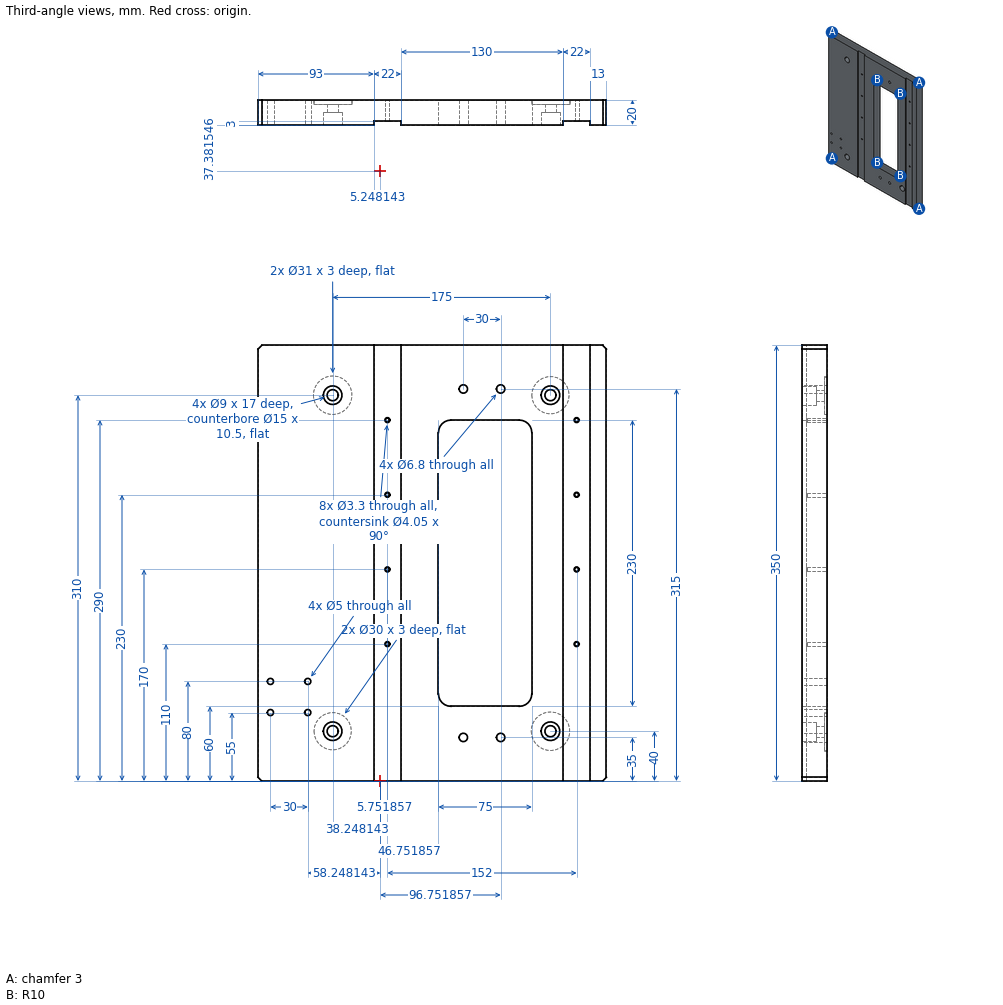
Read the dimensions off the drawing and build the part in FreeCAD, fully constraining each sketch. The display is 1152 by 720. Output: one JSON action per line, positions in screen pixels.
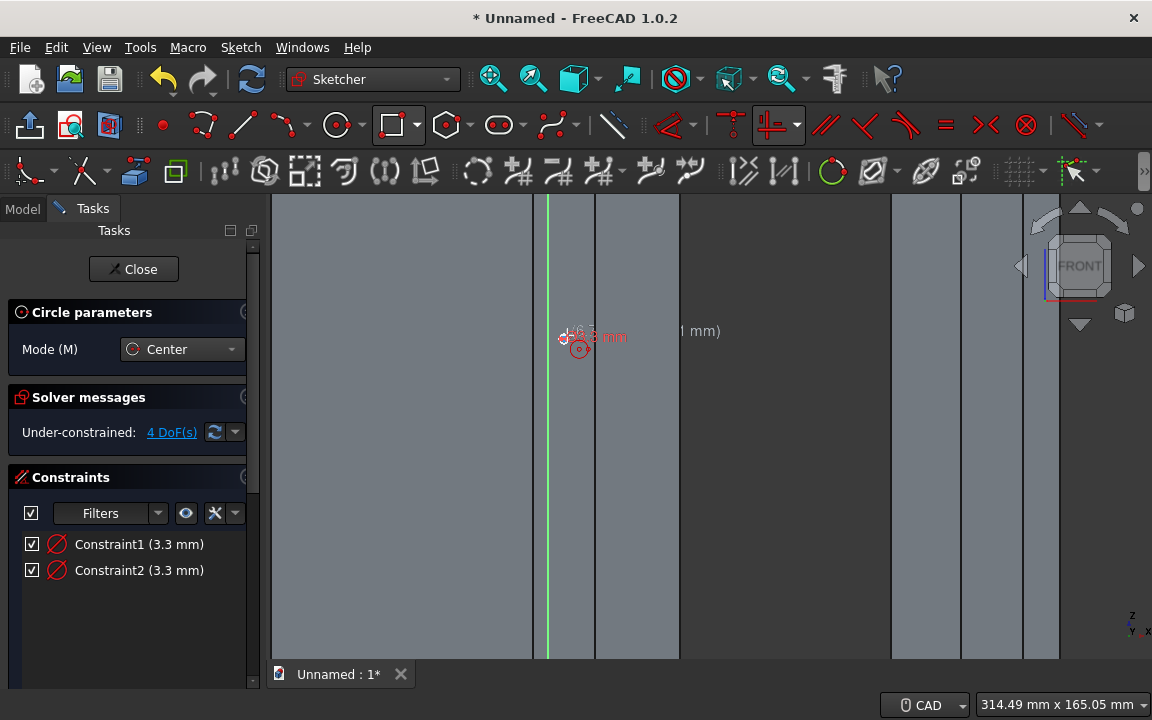
{"action": "scroll", "coordinate": [564, 507], "scroll_direction": "up", "scroll_amount": 8}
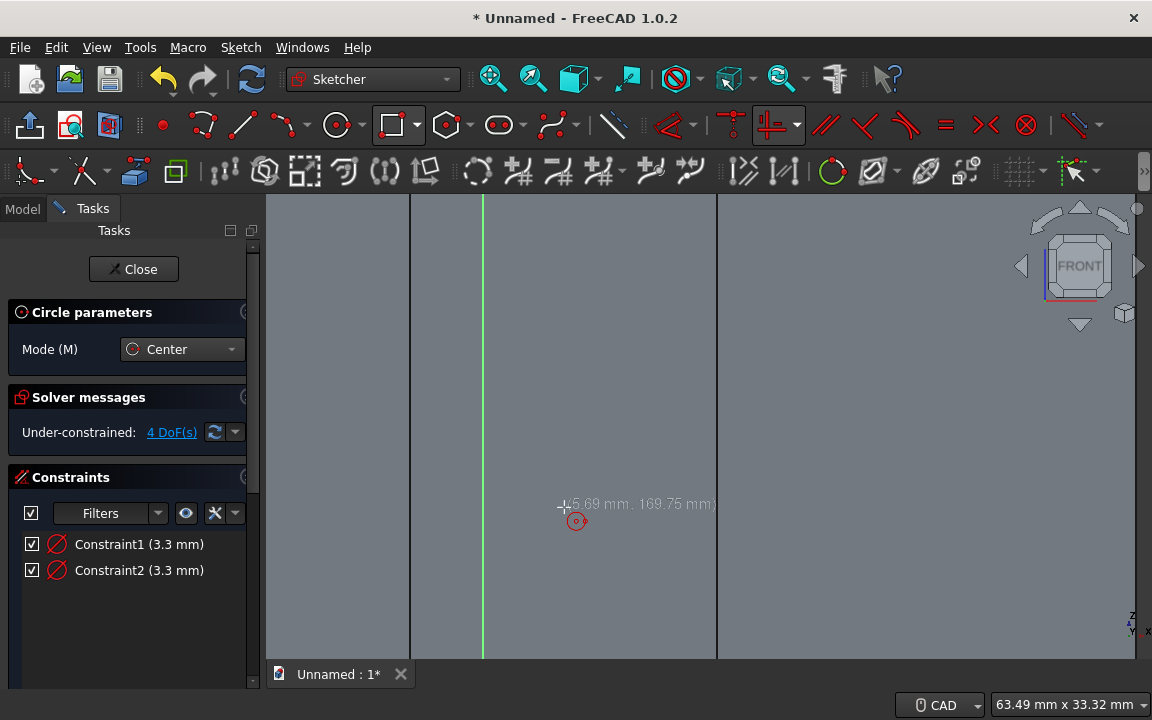
{"action": "scroll", "coordinate": [564, 393], "scroll_direction": "down", "scroll_amount": 13}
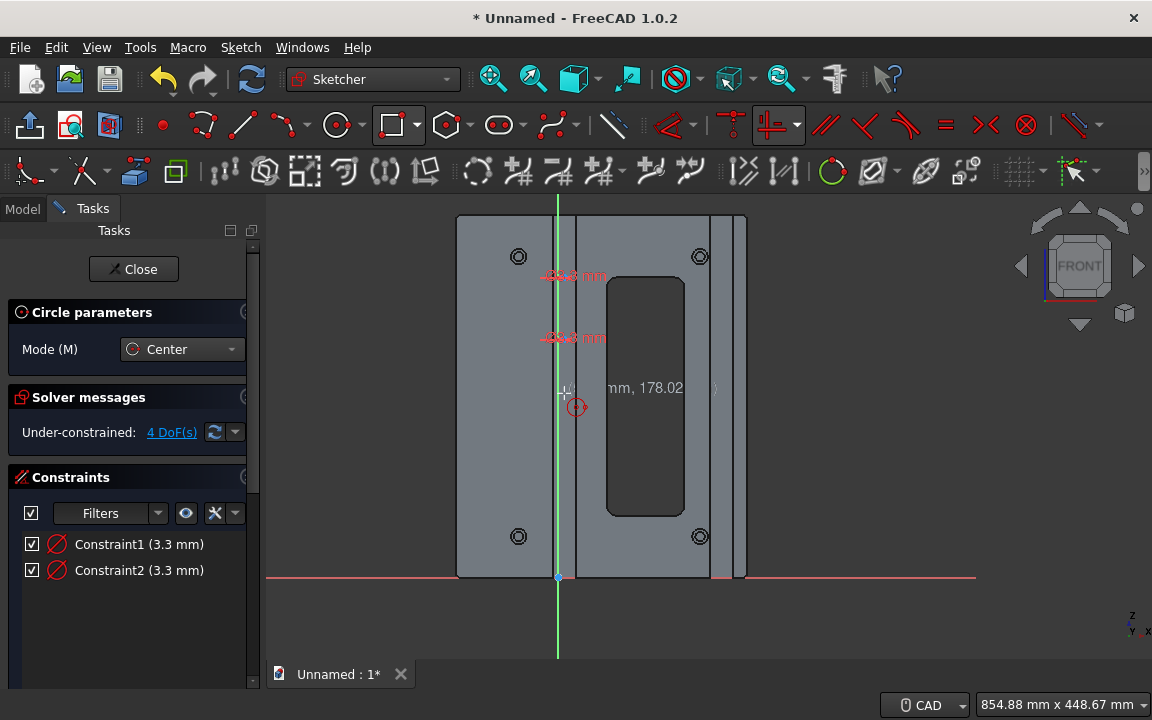
{"action": "scroll", "coordinate": [564, 402], "scroll_direction": "up", "scroll_amount": 5}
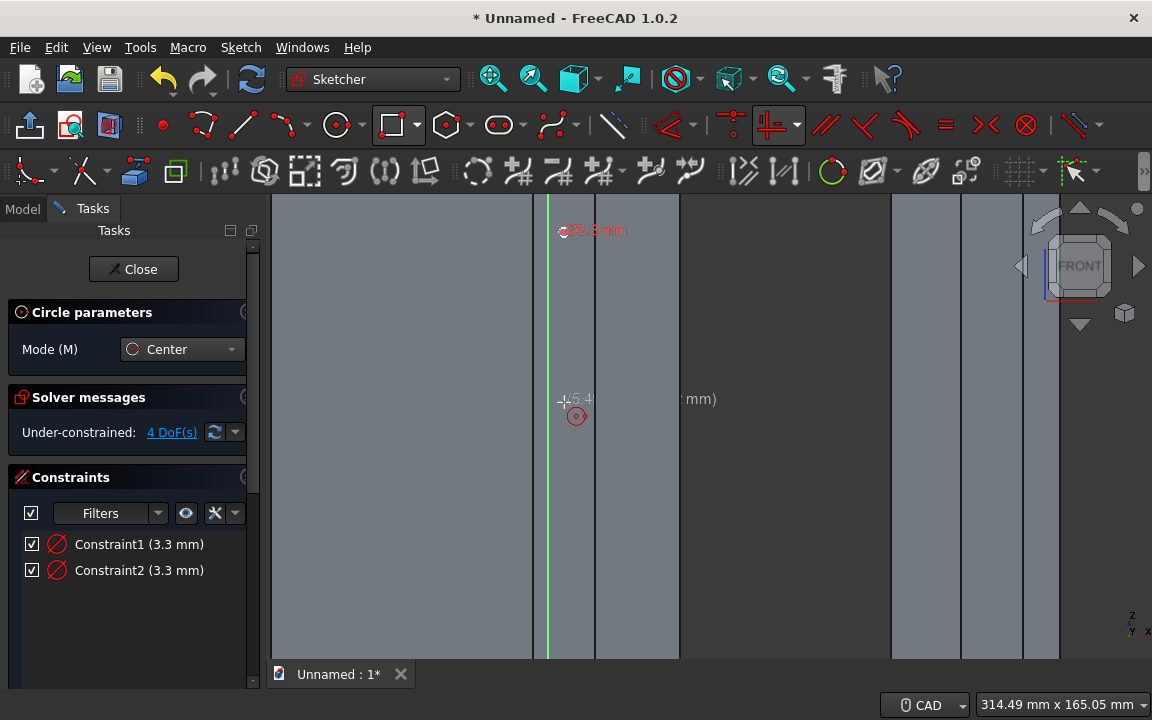
{"action": "left_click", "coordinate": [564, 401]}
{"action": "mouse_move", "coordinate": [567, 397]}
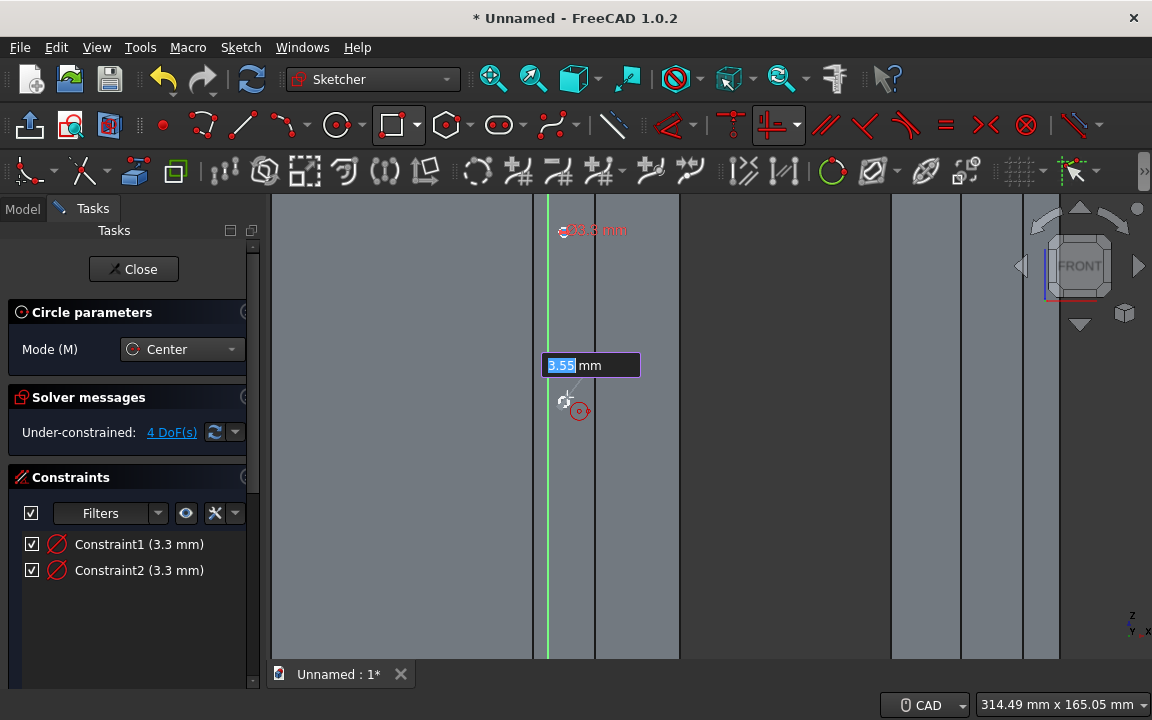
{"action": "type", "text": "3.3"}
{"action": "key", "text": "Return"}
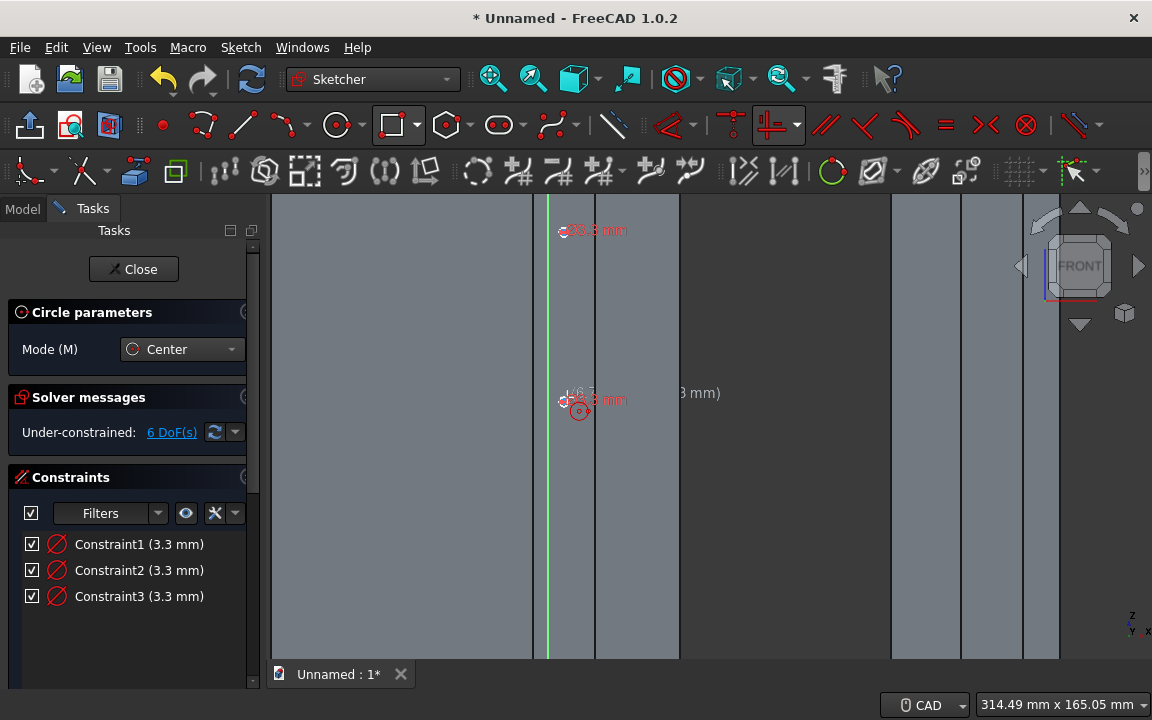
{"action": "scroll", "coordinate": [564, 402], "scroll_direction": "down", "scroll_amount": 5}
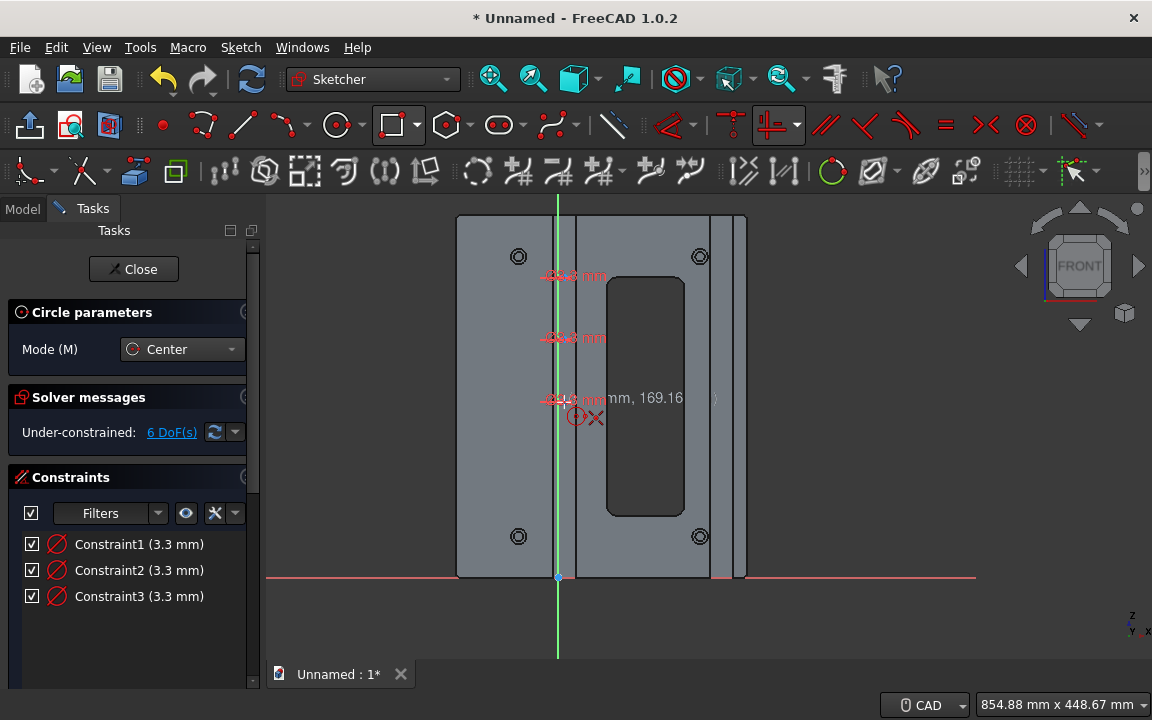
{"action": "scroll", "coordinate": [722, 402], "scroll_direction": "up", "scroll_amount": 13}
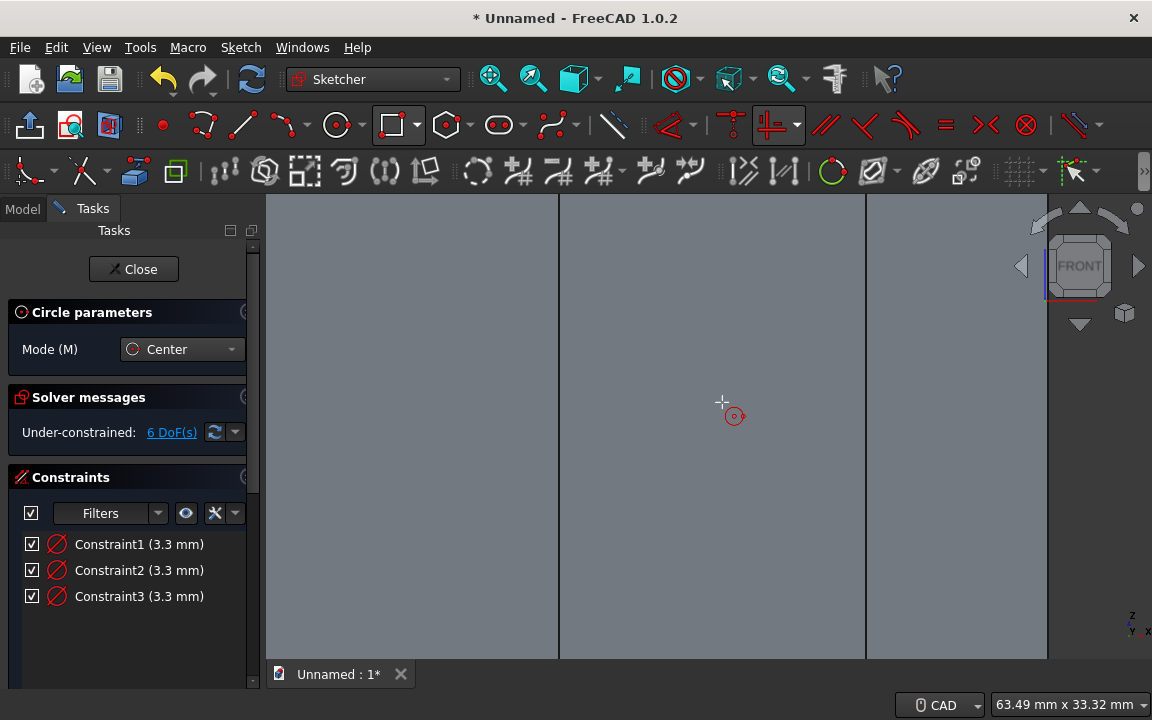
{"action": "scroll", "coordinate": [722, 402], "scroll_direction": "down", "scroll_amount": 13}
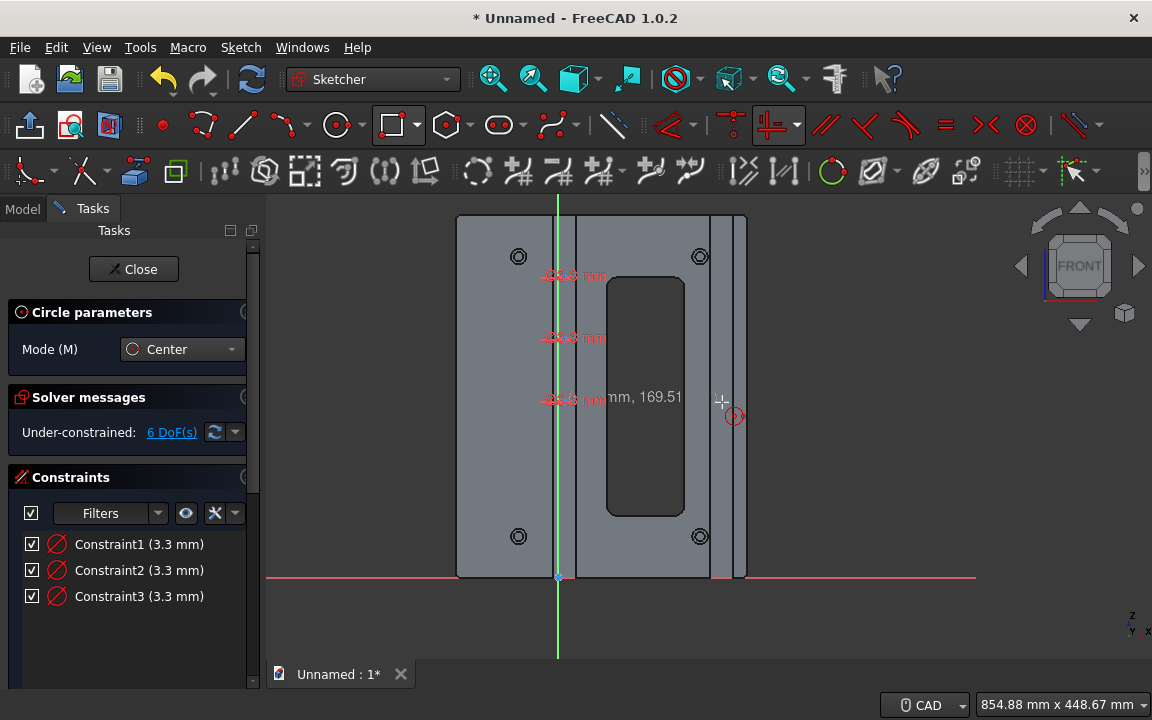
{"action": "left_click", "coordinate": [722, 402]}
{"action": "mouse_move", "coordinate": [723, 401]}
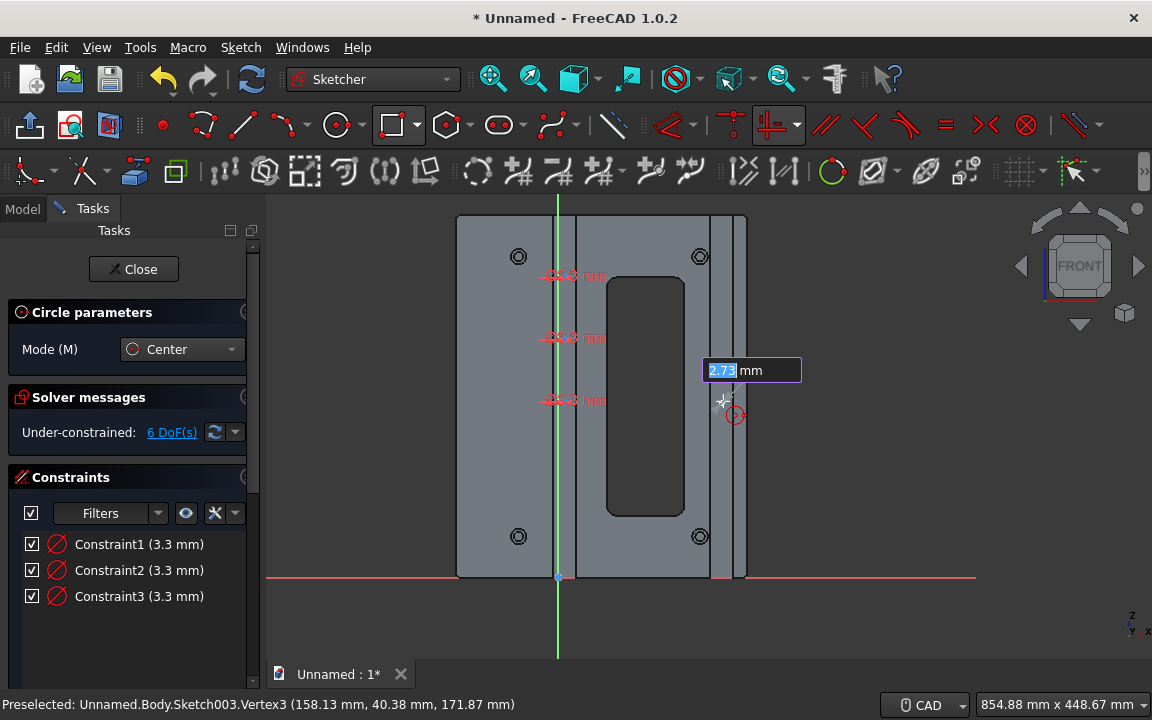
{"action": "type", "text": "3.3"}
{"action": "key", "text": "Return"}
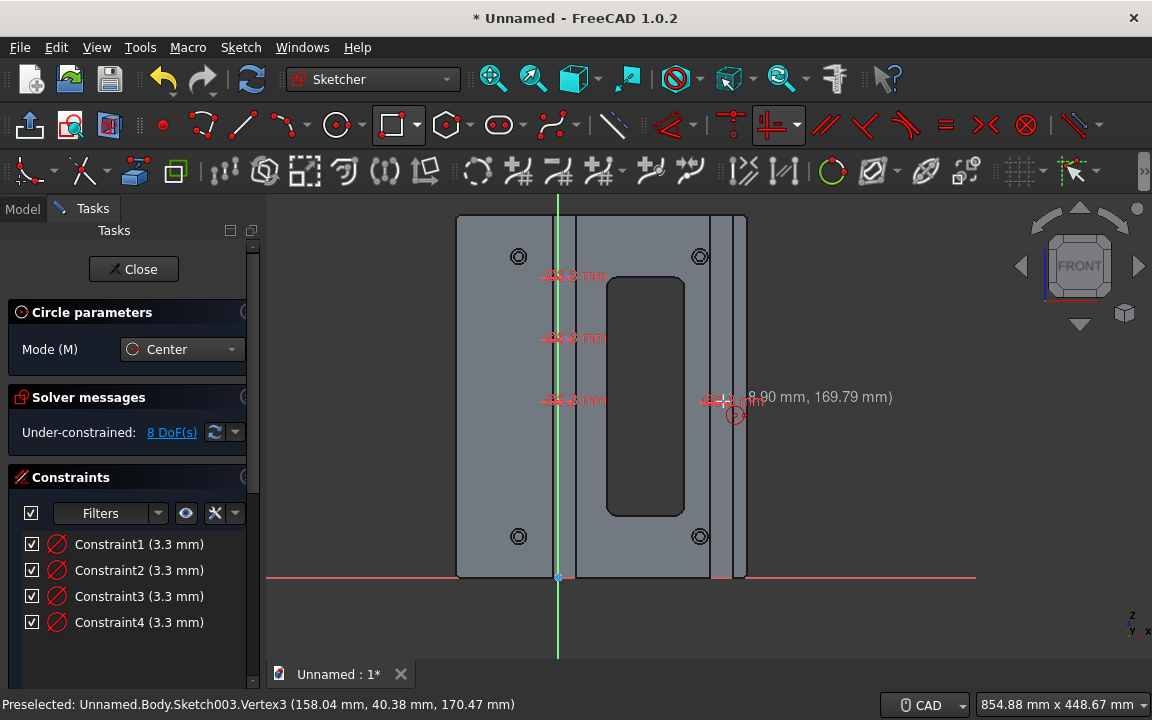
{"action": "scroll", "coordinate": [722, 340], "scroll_direction": "up", "scroll_amount": 13}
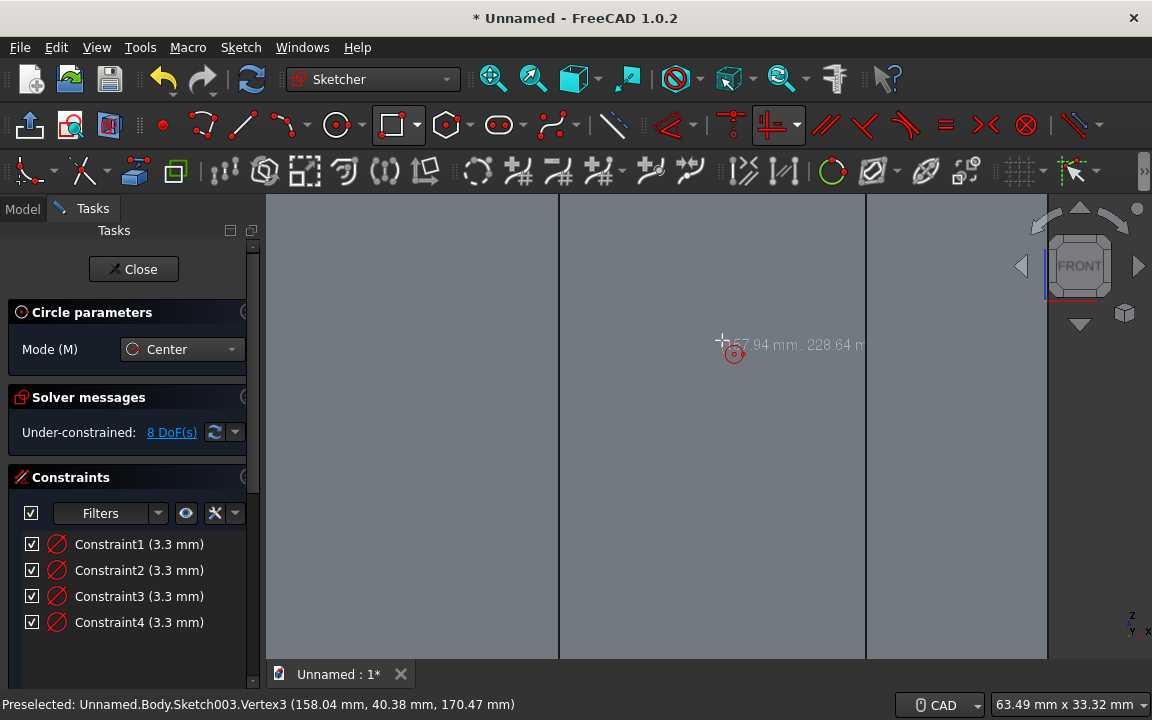
{"action": "scroll", "coordinate": [722, 340], "scroll_direction": "down", "scroll_amount": 13}